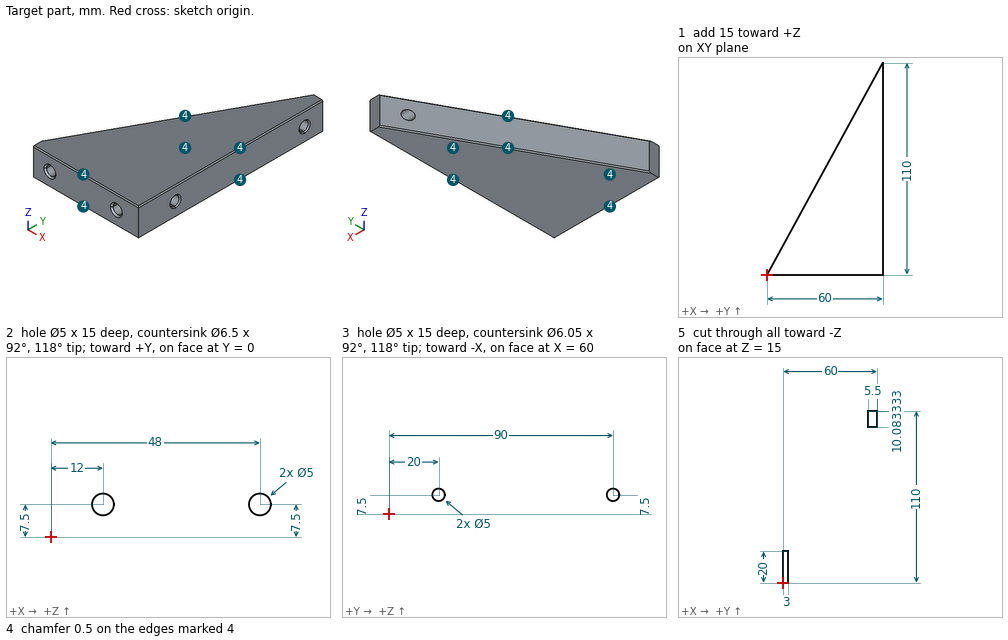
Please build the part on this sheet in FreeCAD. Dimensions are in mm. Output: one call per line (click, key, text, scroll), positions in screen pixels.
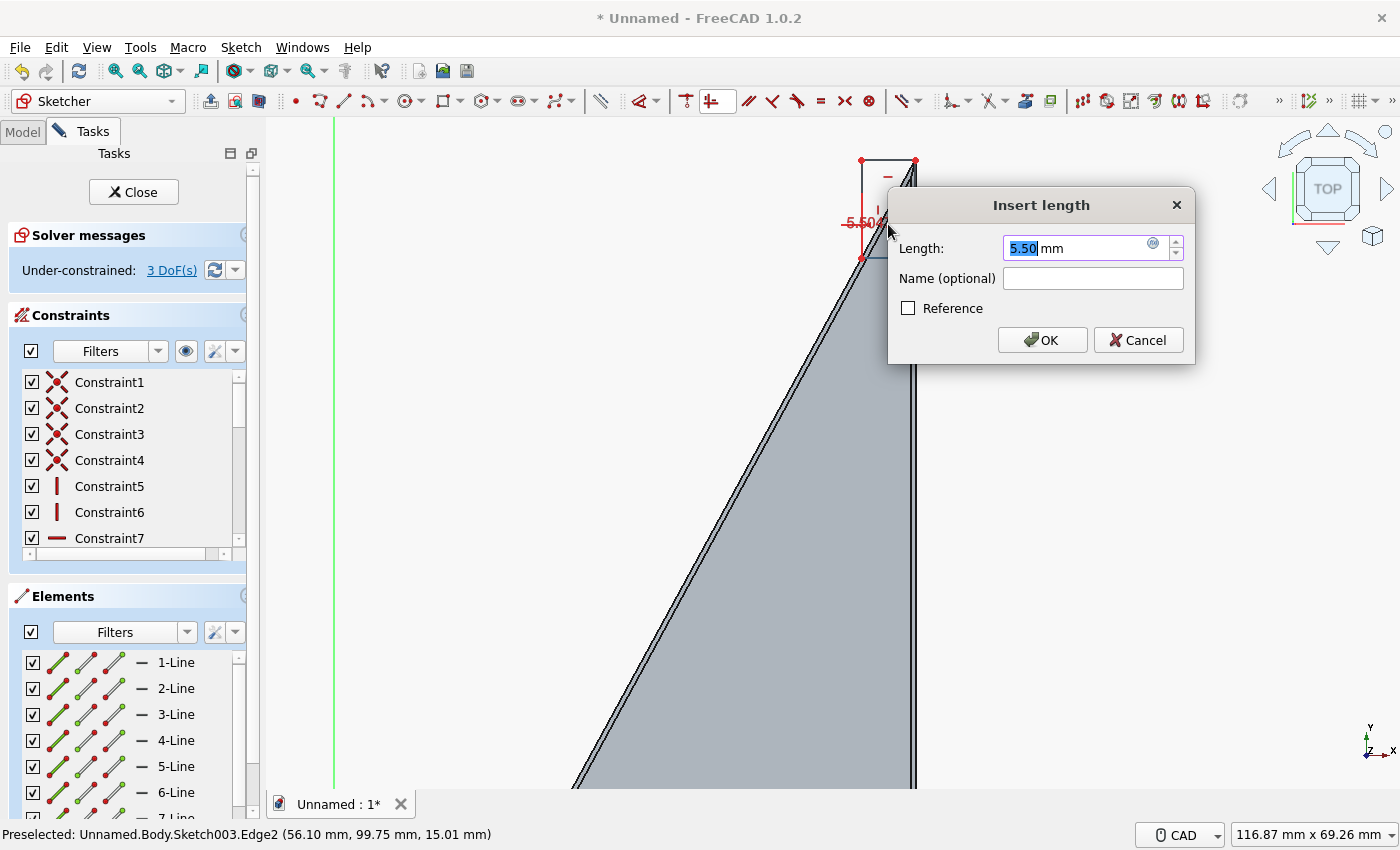
text(5.5)
key(Return)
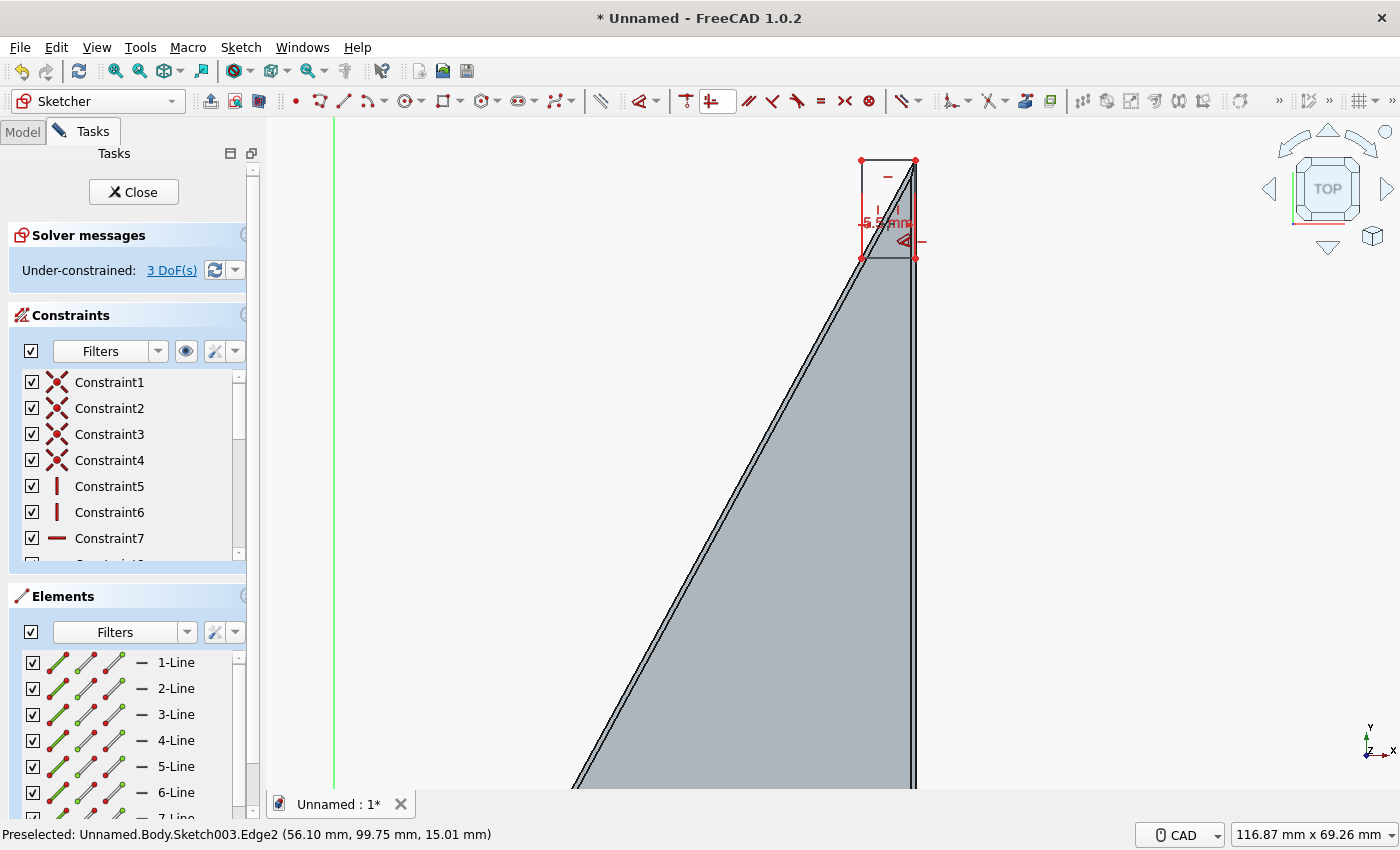
click(915, 258)
click(624, 224)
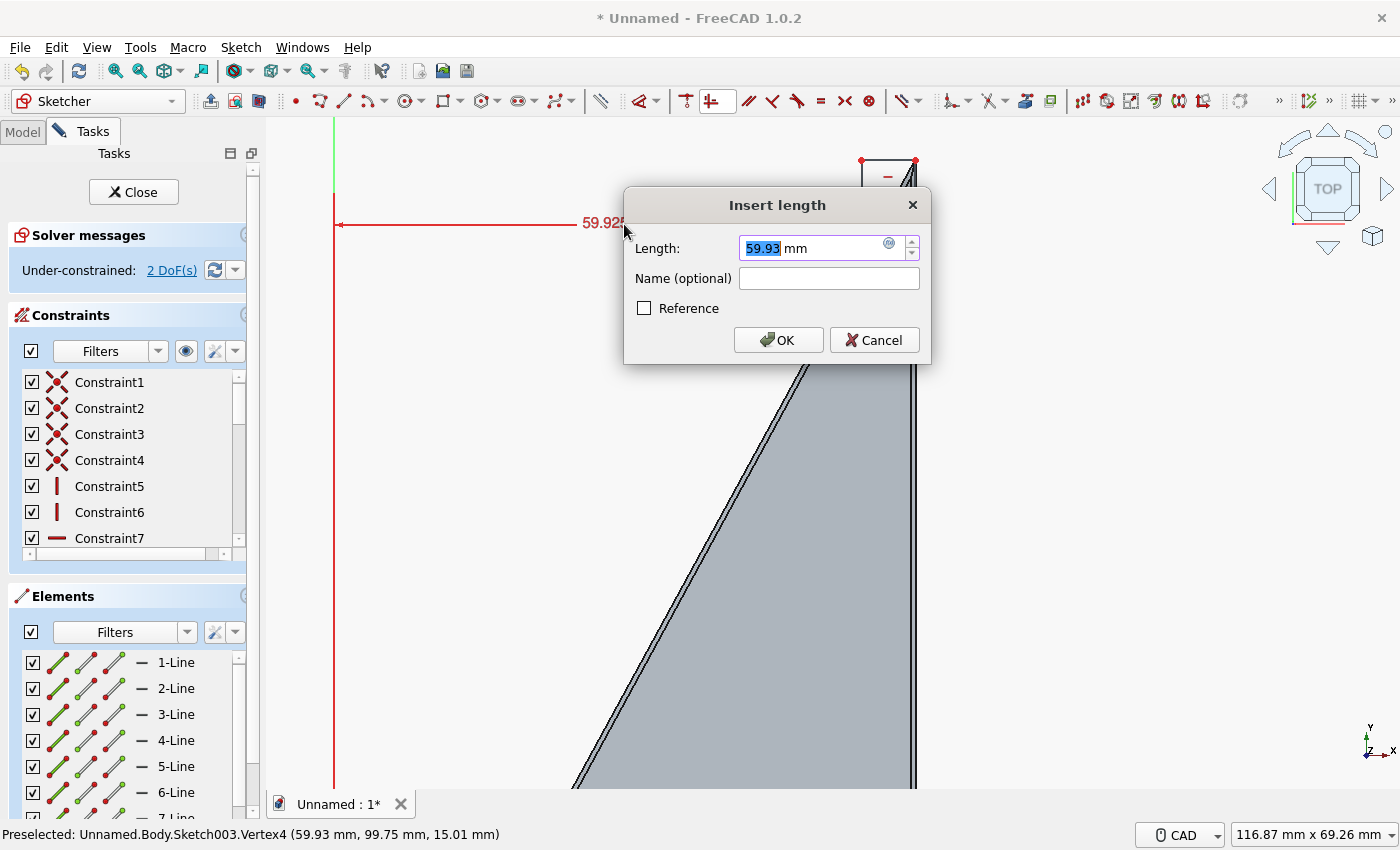
text(60)
key(Return)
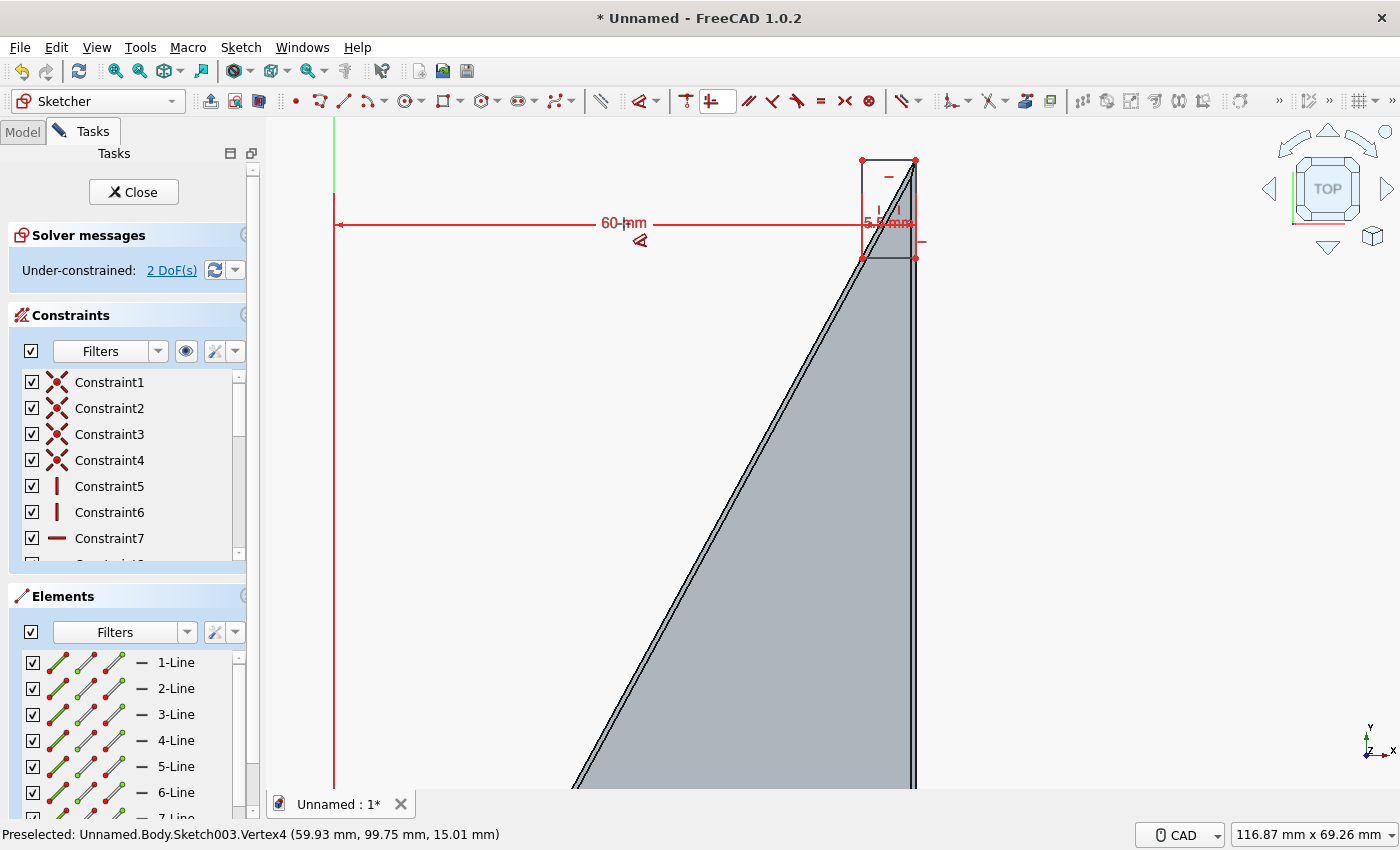
click(862, 160)
click(300, 461)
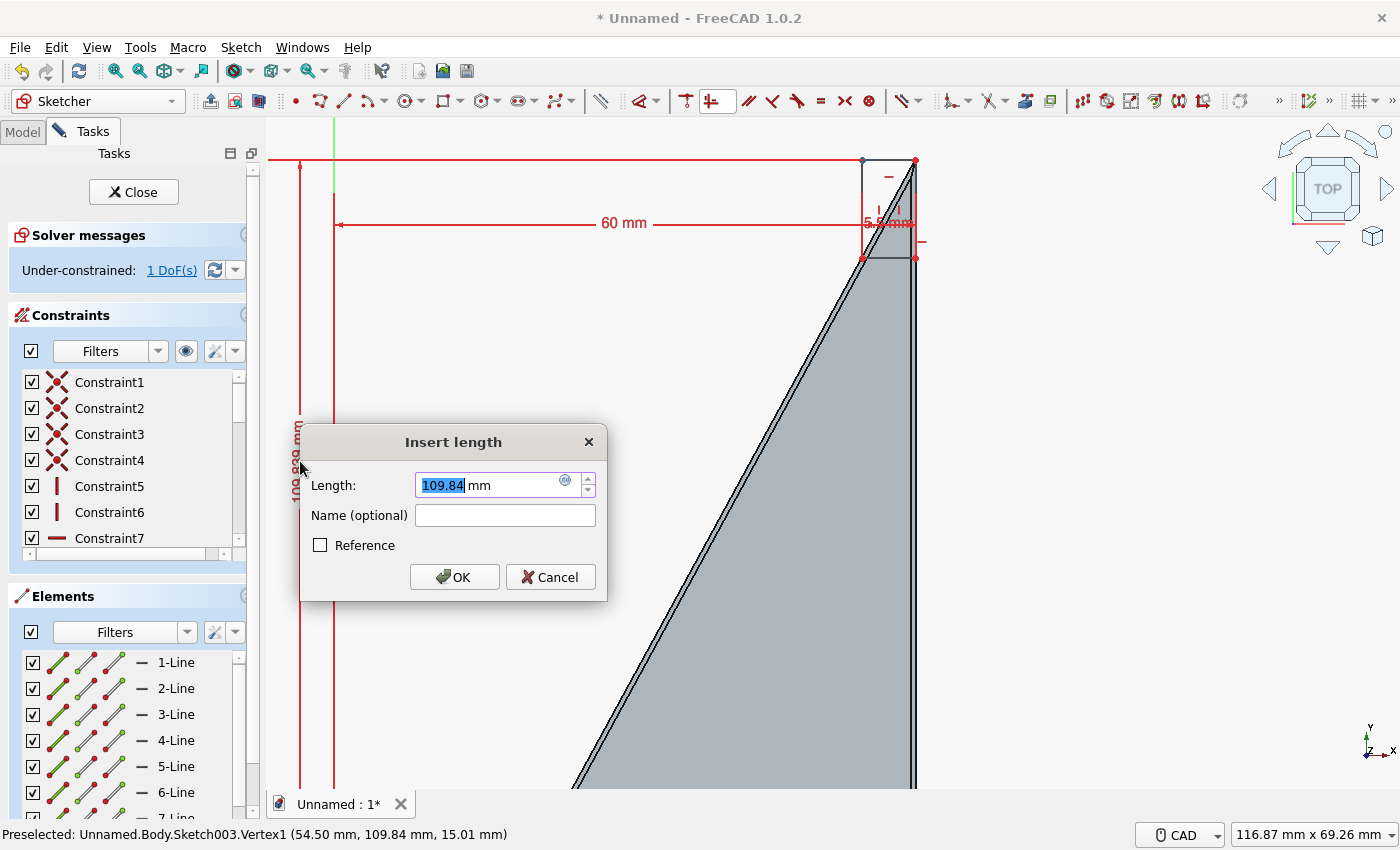
text(110)
key(Return)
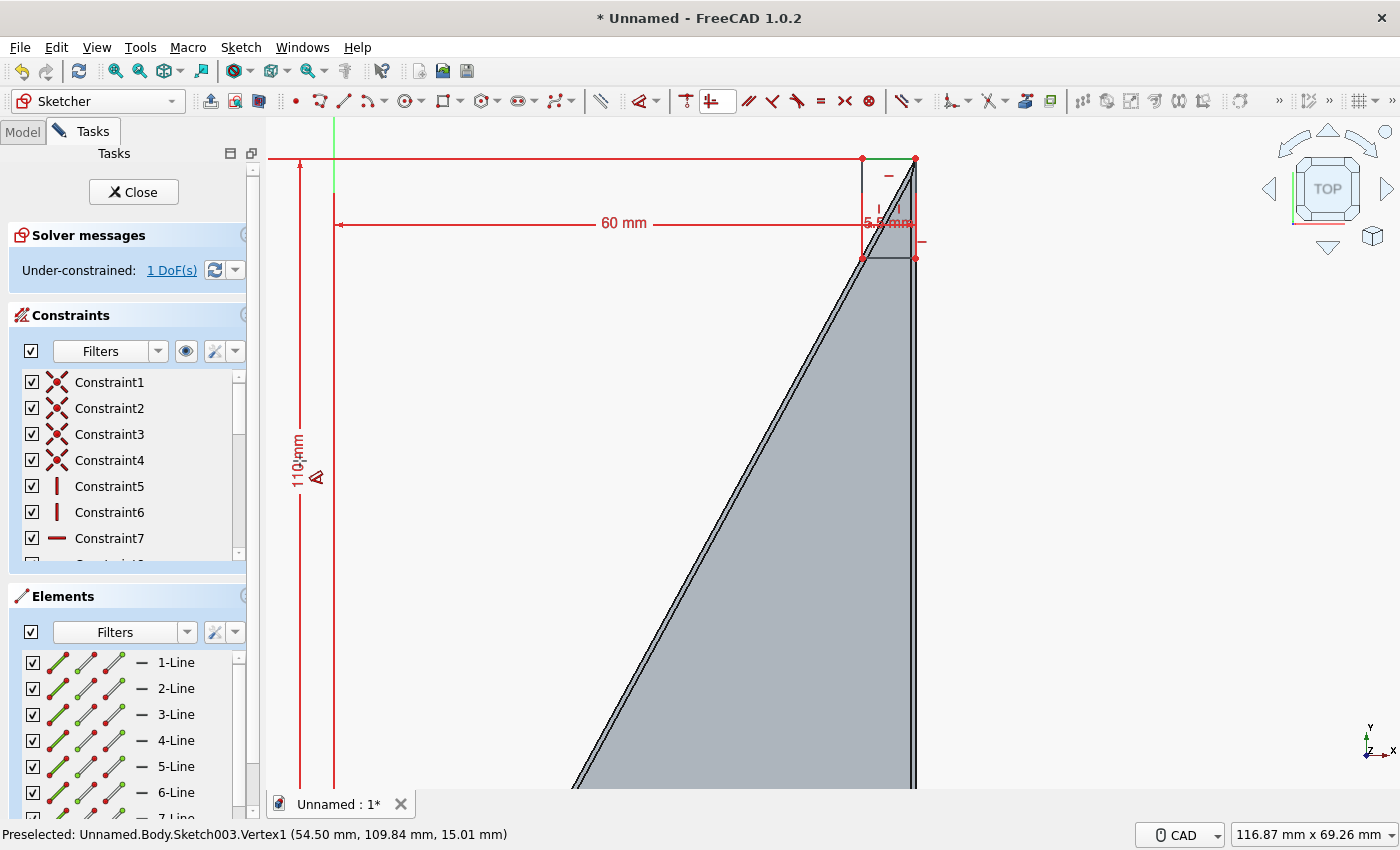
click(862, 188)
click(896, 185)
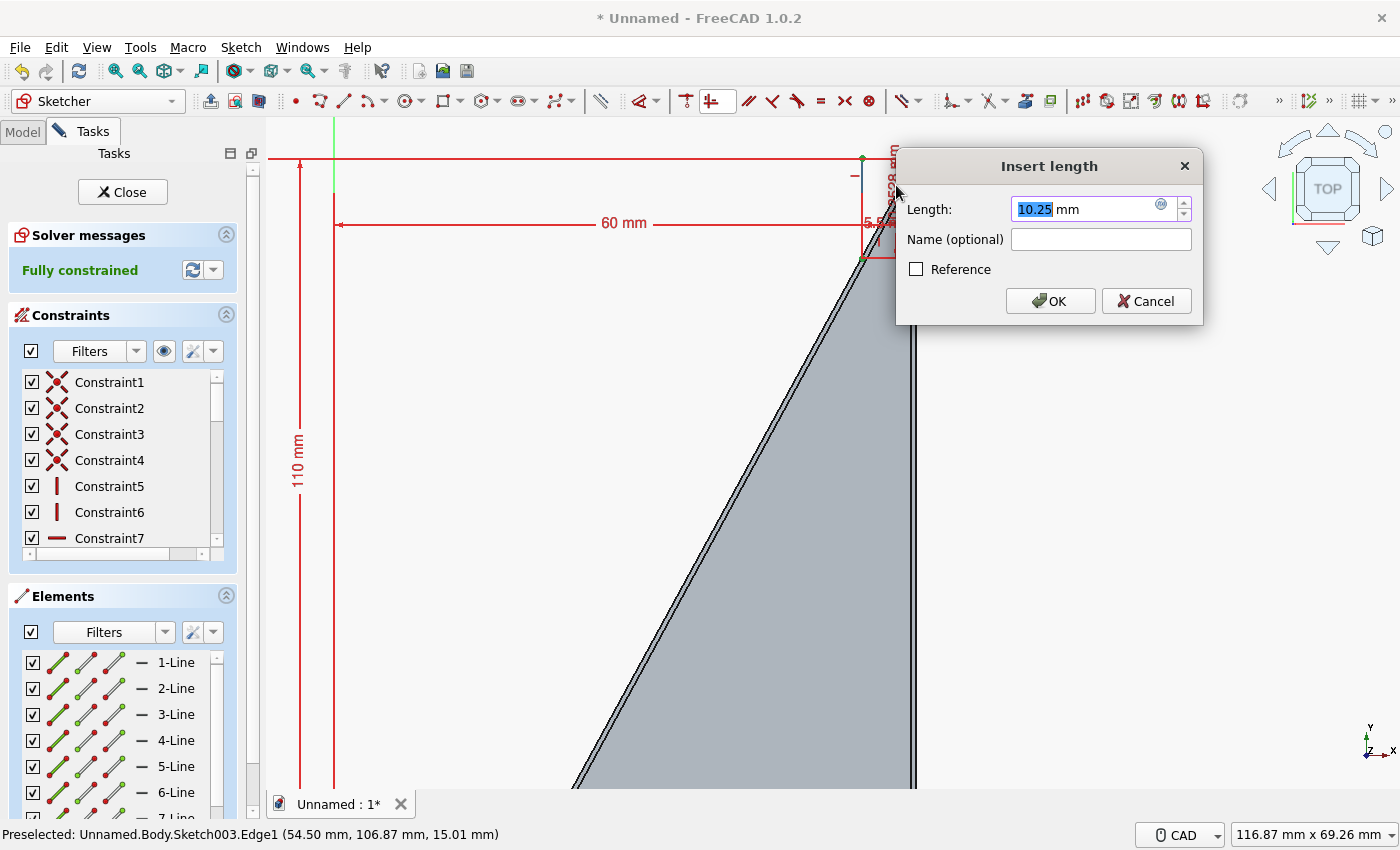
text(10.083333)
key(Return)
key(Escape)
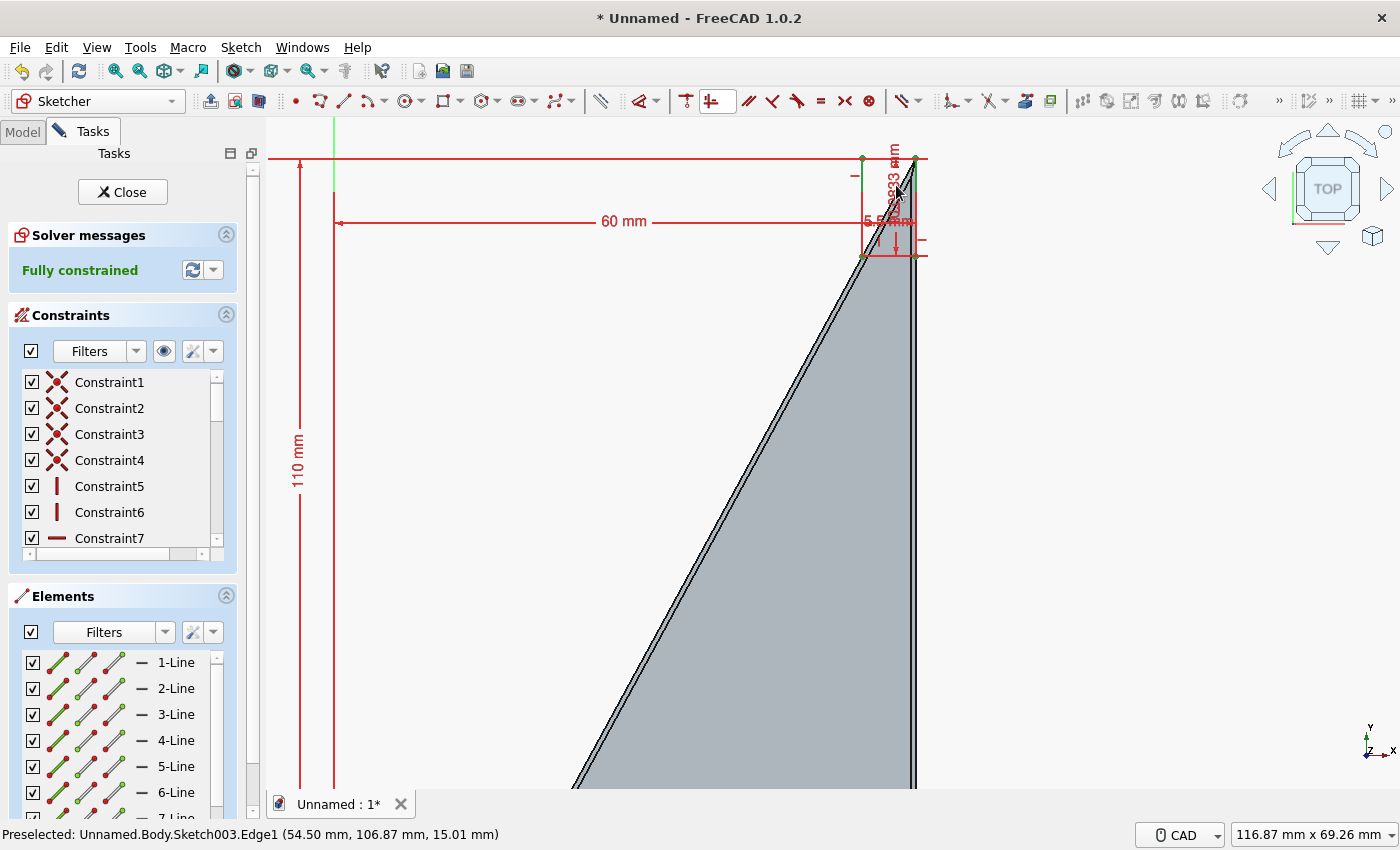
click(123, 192)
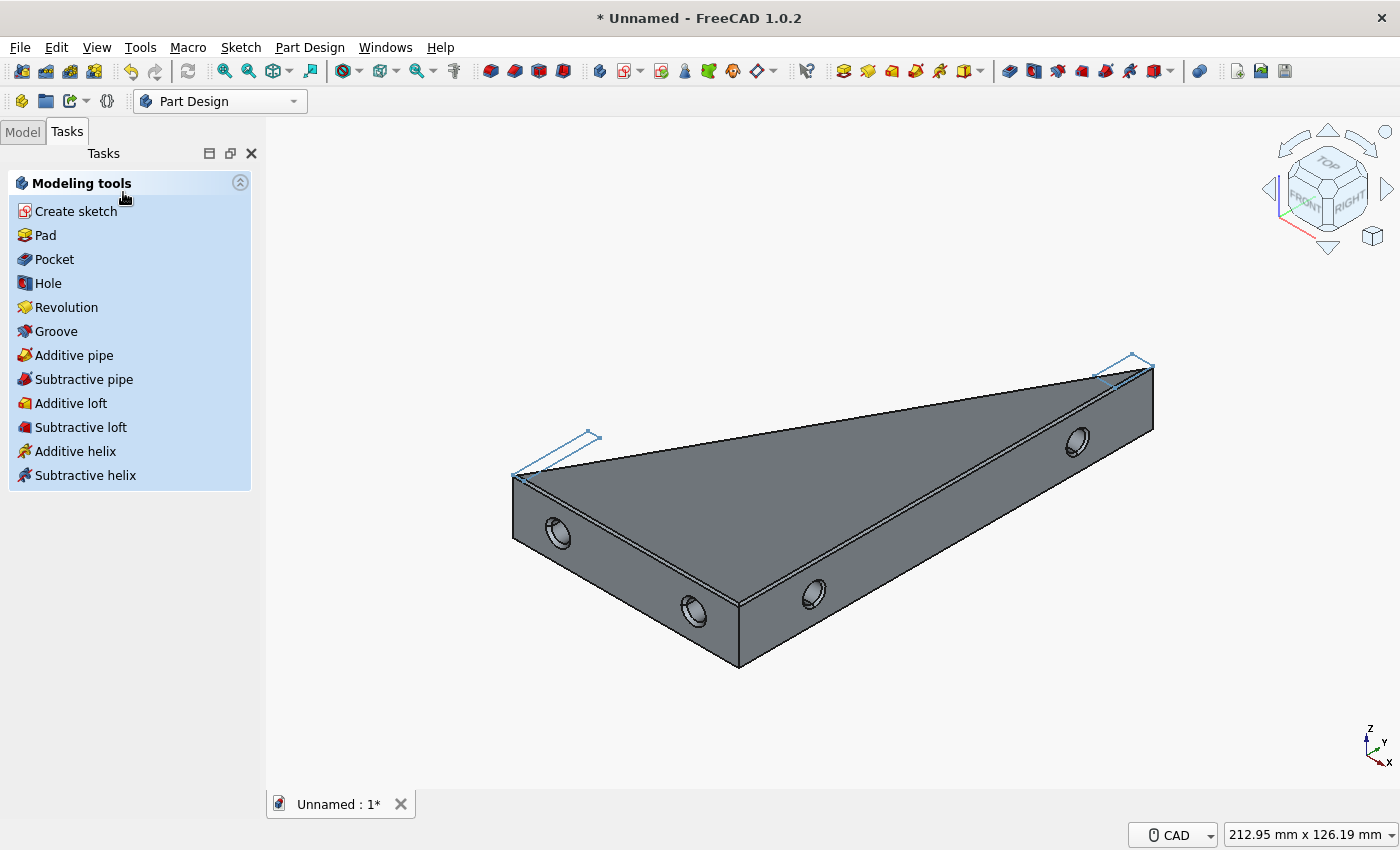
click(1010, 72)